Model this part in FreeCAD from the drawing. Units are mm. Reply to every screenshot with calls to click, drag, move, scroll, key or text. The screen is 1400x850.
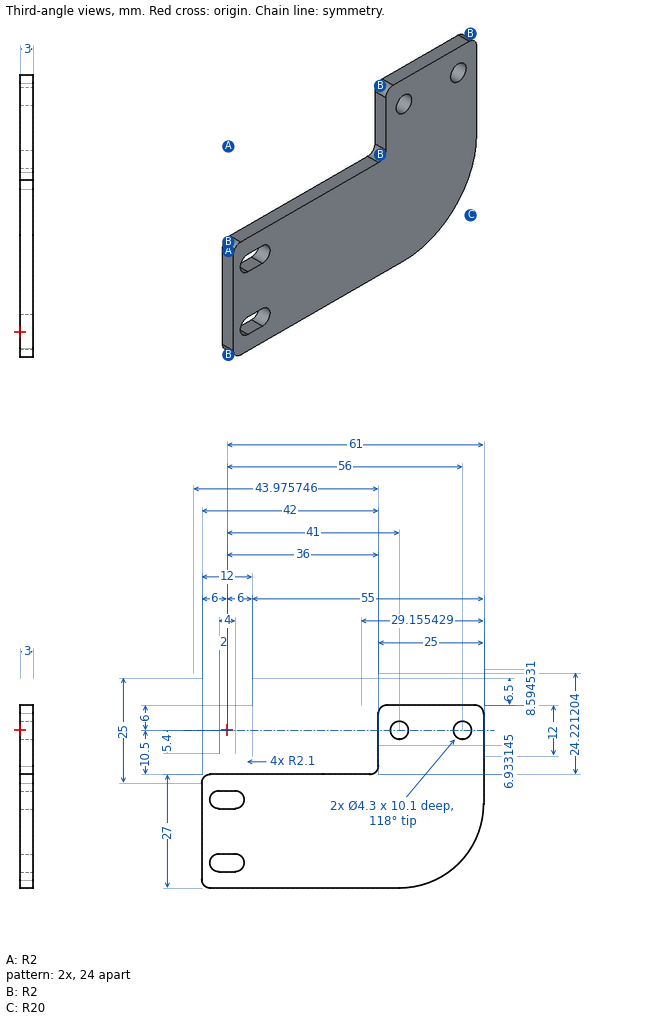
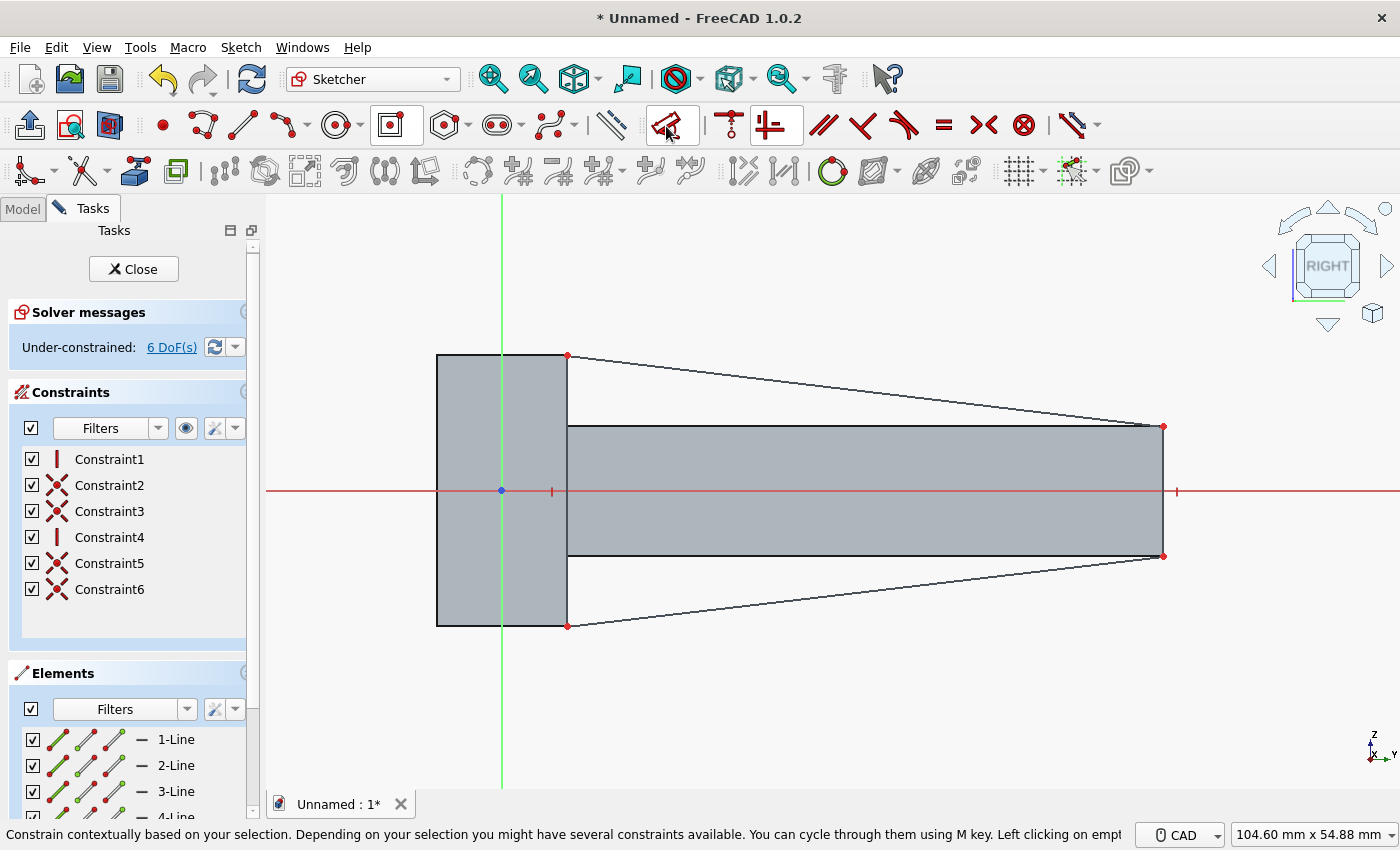
click(567, 546)
click(533, 429)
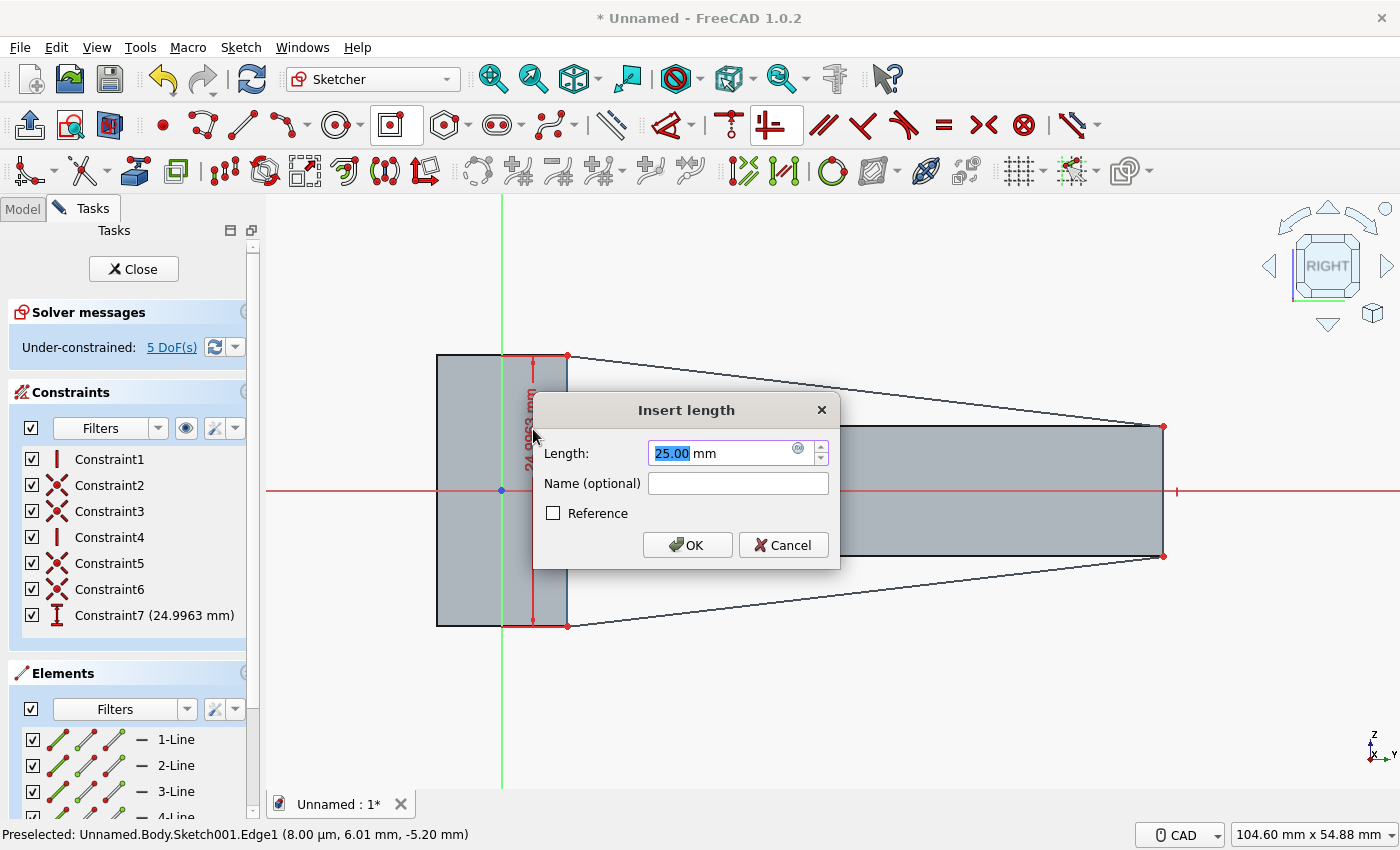
text(25)
key(Return)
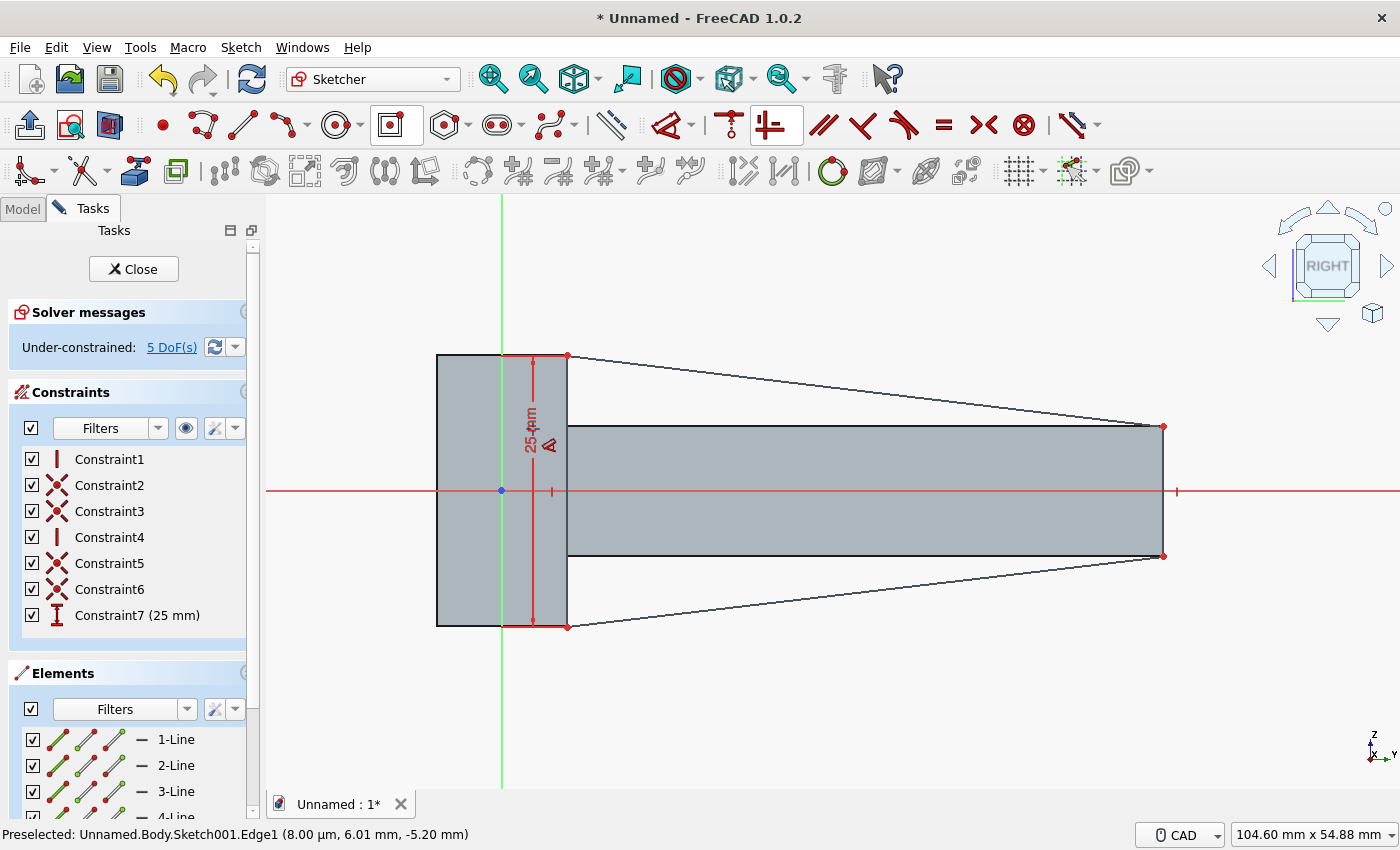
click(1163, 466)
click(1197, 462)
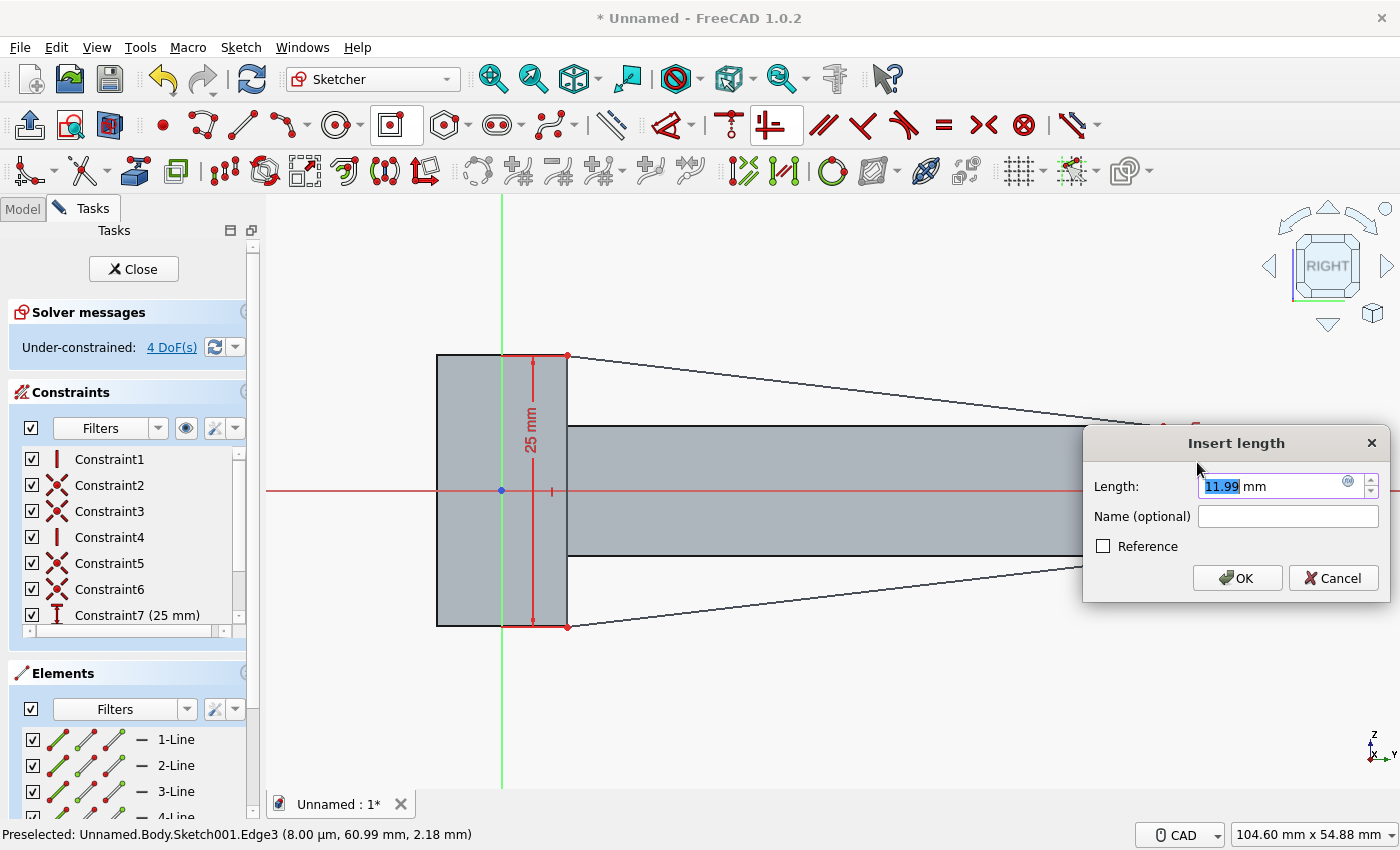
text(12)
key(Return)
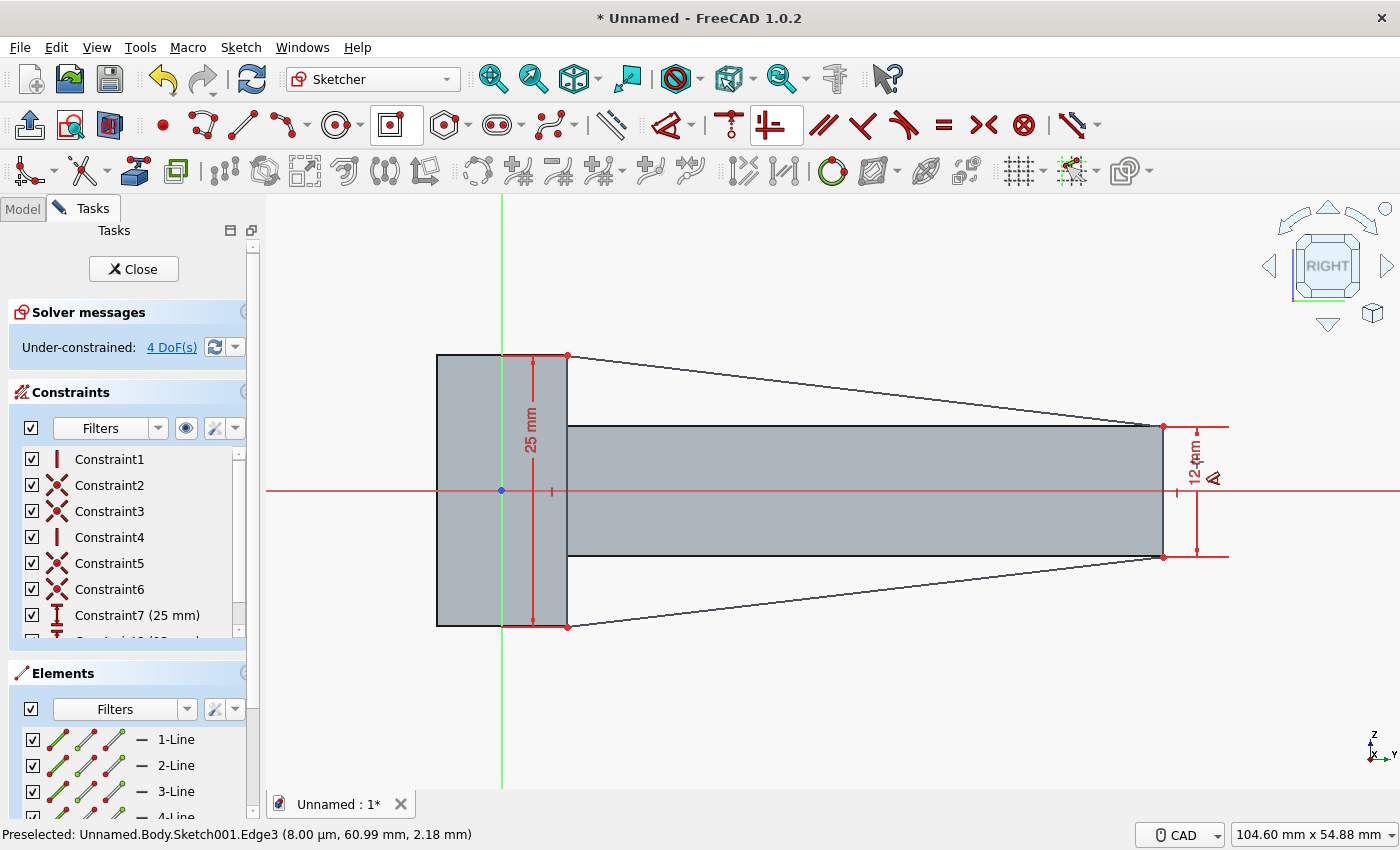
click(567, 627)
click(534, 661)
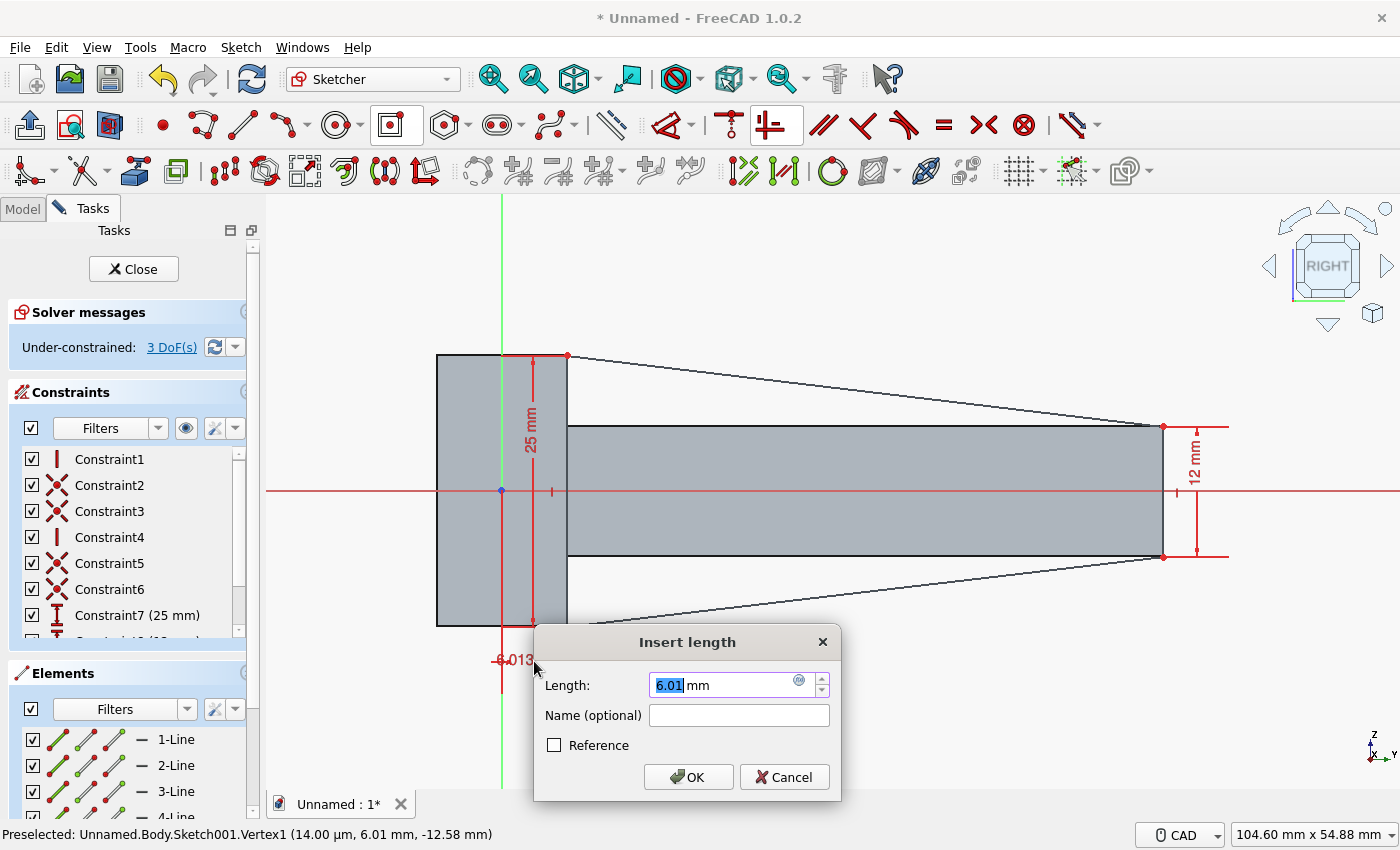
text(6)
key(Return)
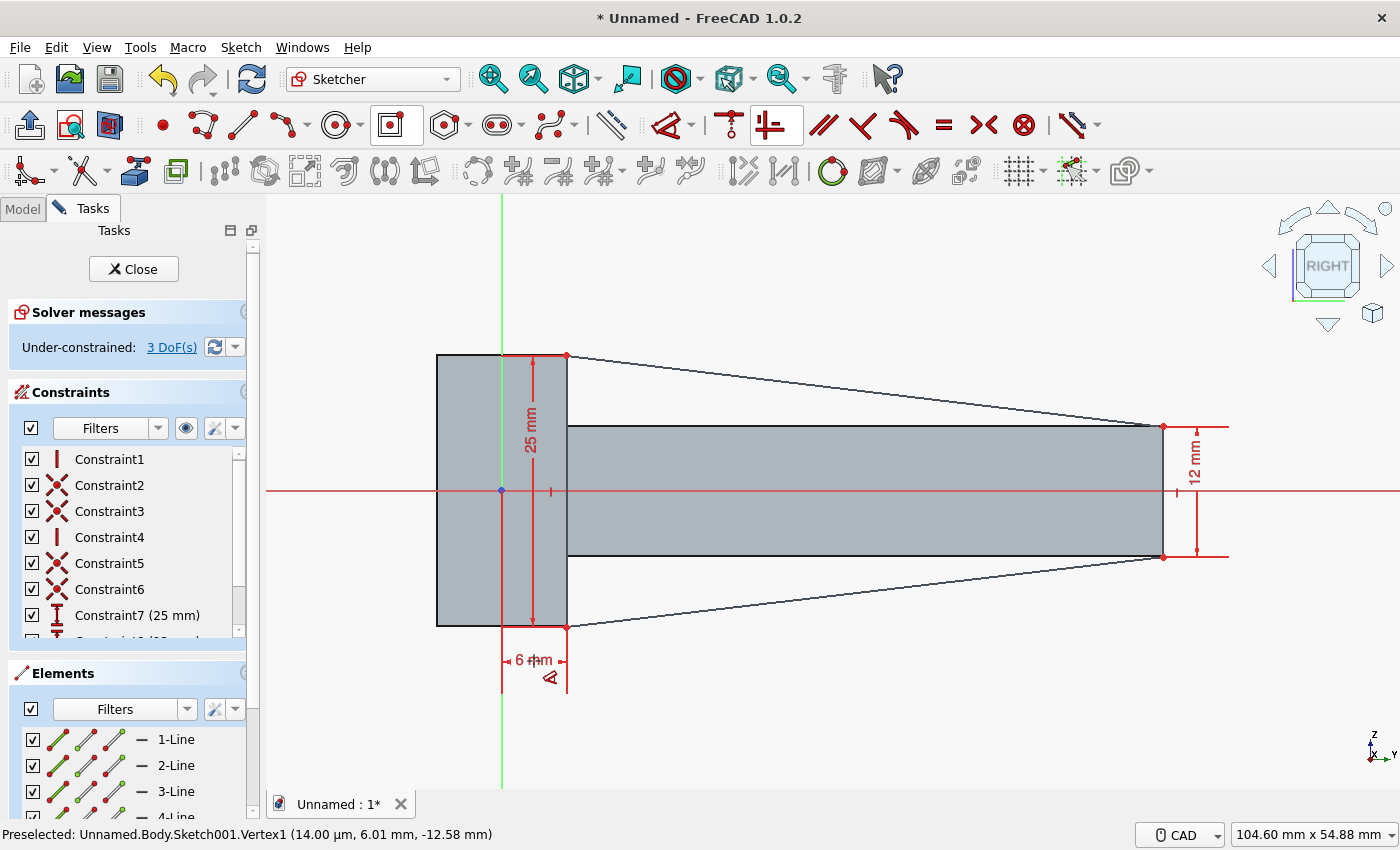
click(1163, 427)
click(468, 459)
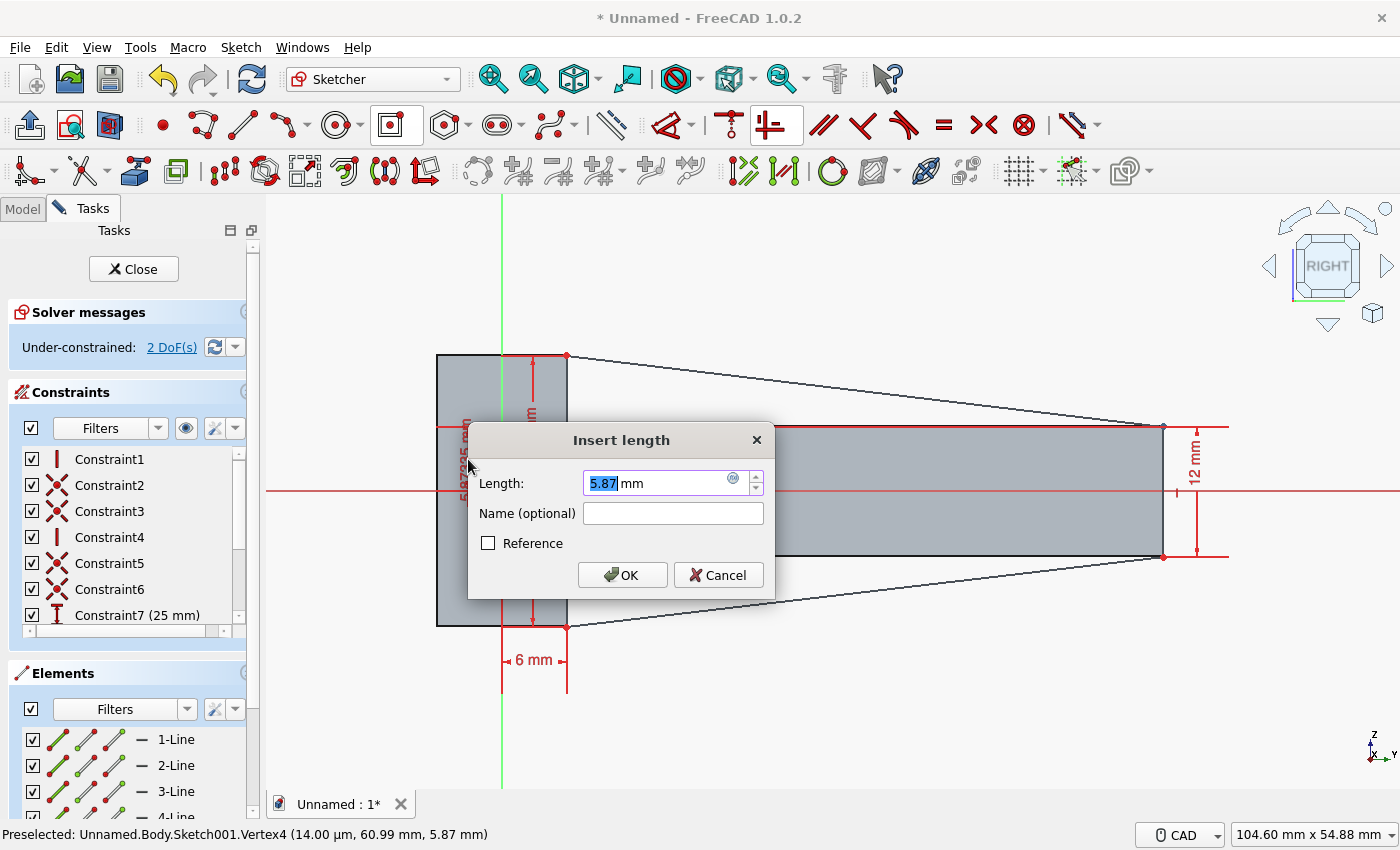
text(6)
key(Return)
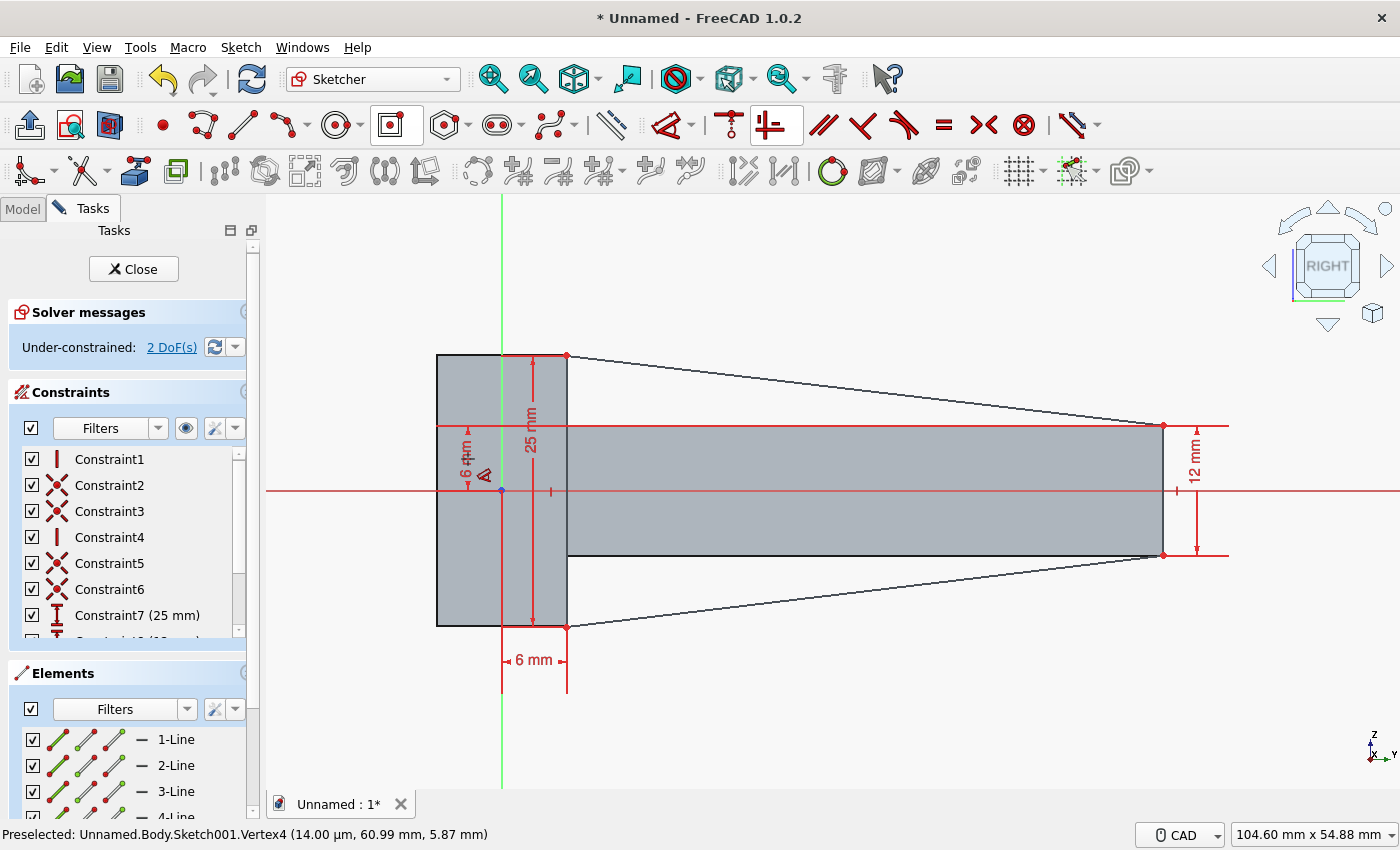
click(1163, 426)
click(680, 392)